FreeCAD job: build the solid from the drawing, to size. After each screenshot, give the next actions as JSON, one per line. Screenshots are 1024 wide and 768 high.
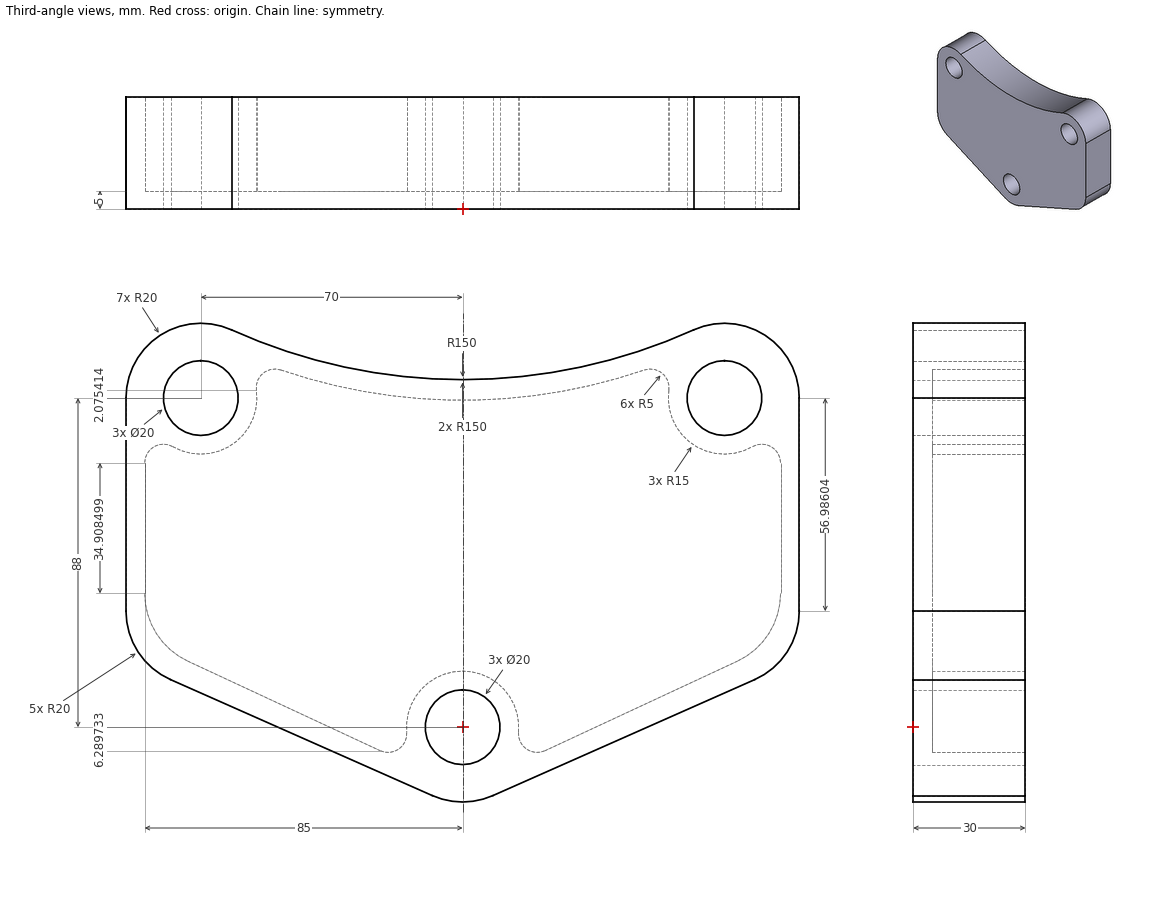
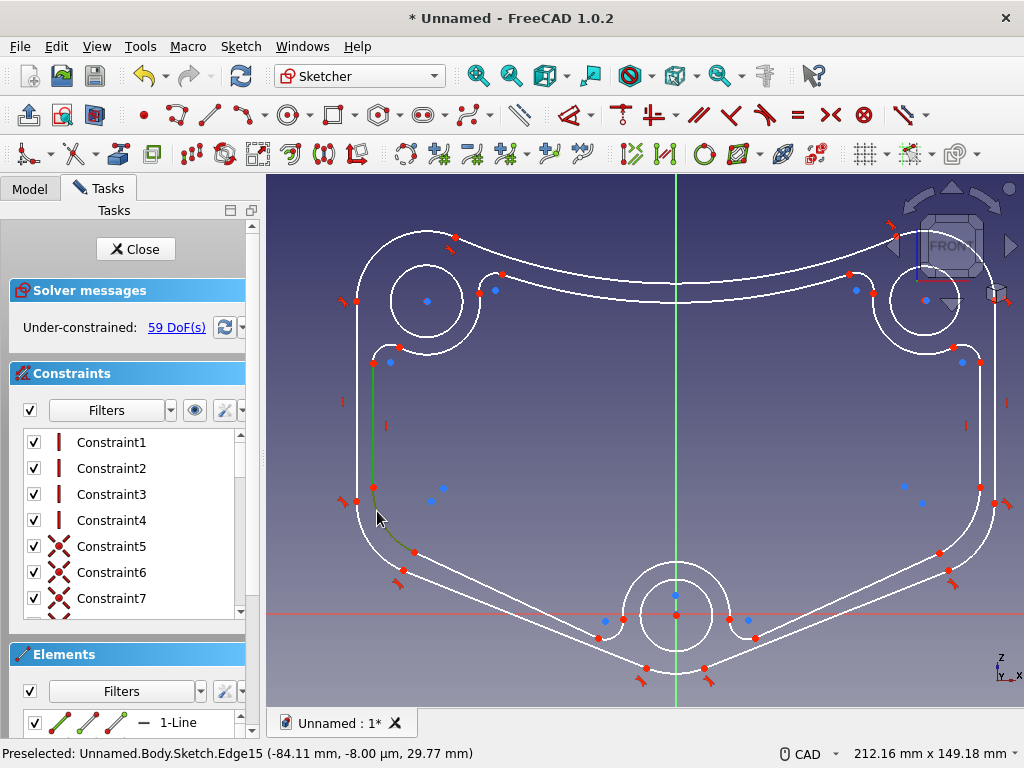
{"action": "left_click", "coordinate": [765, 116]}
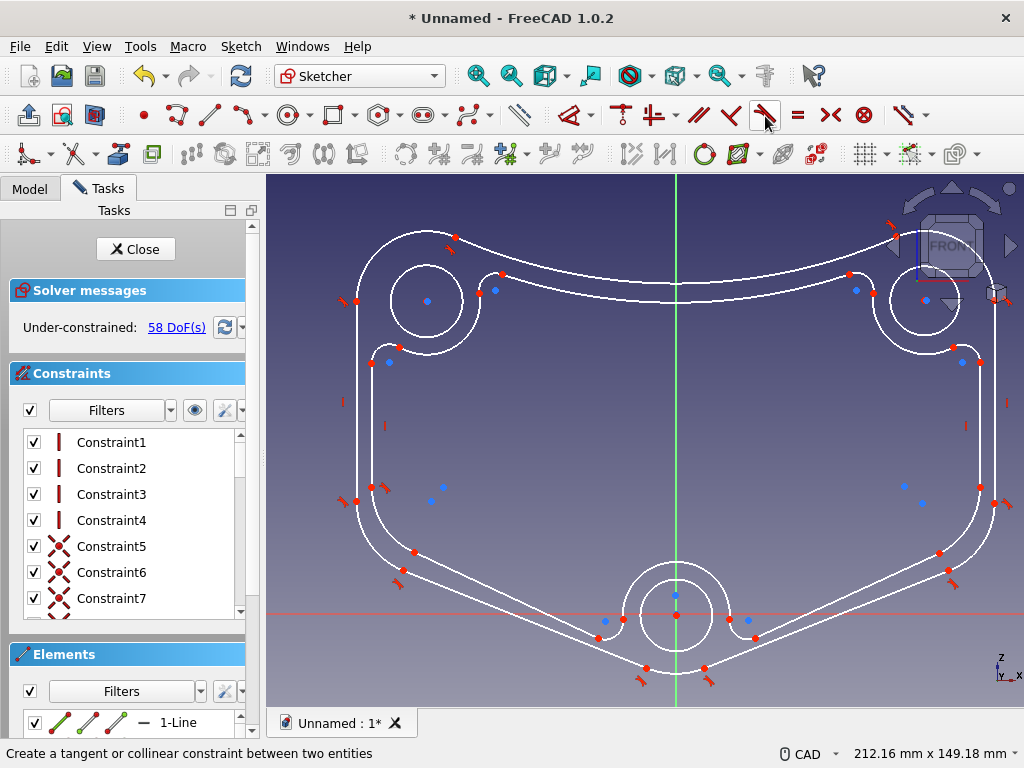
{"action": "left_click", "coordinate": [372, 400]}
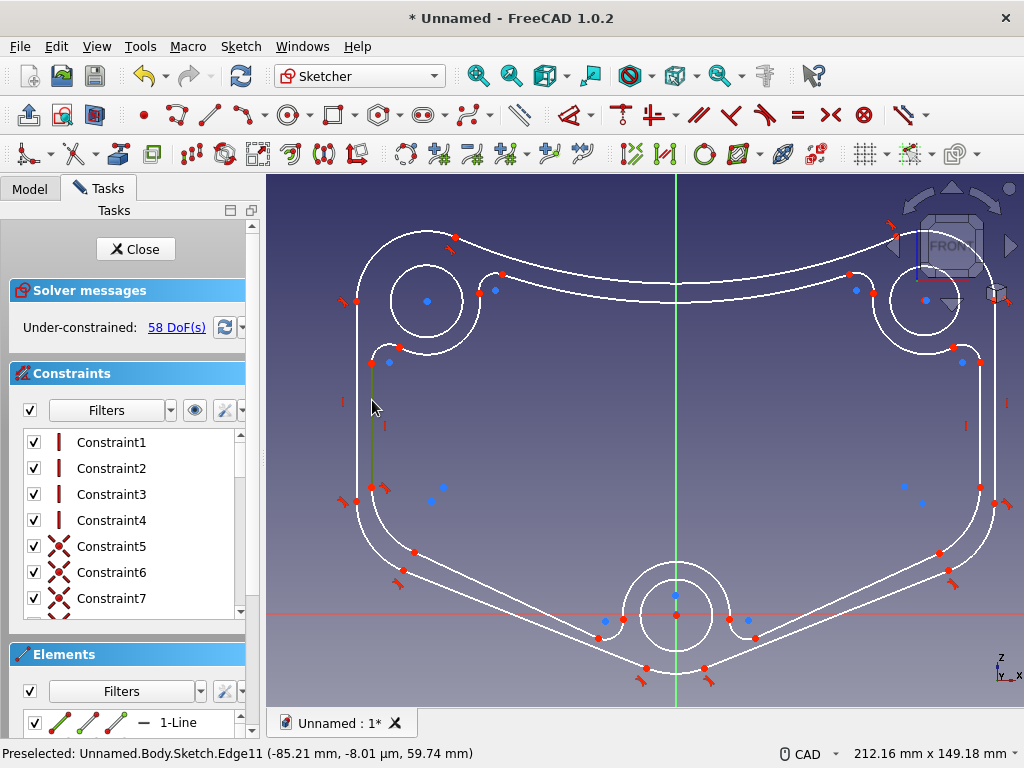
{"action": "left_click", "coordinate": [388, 344]}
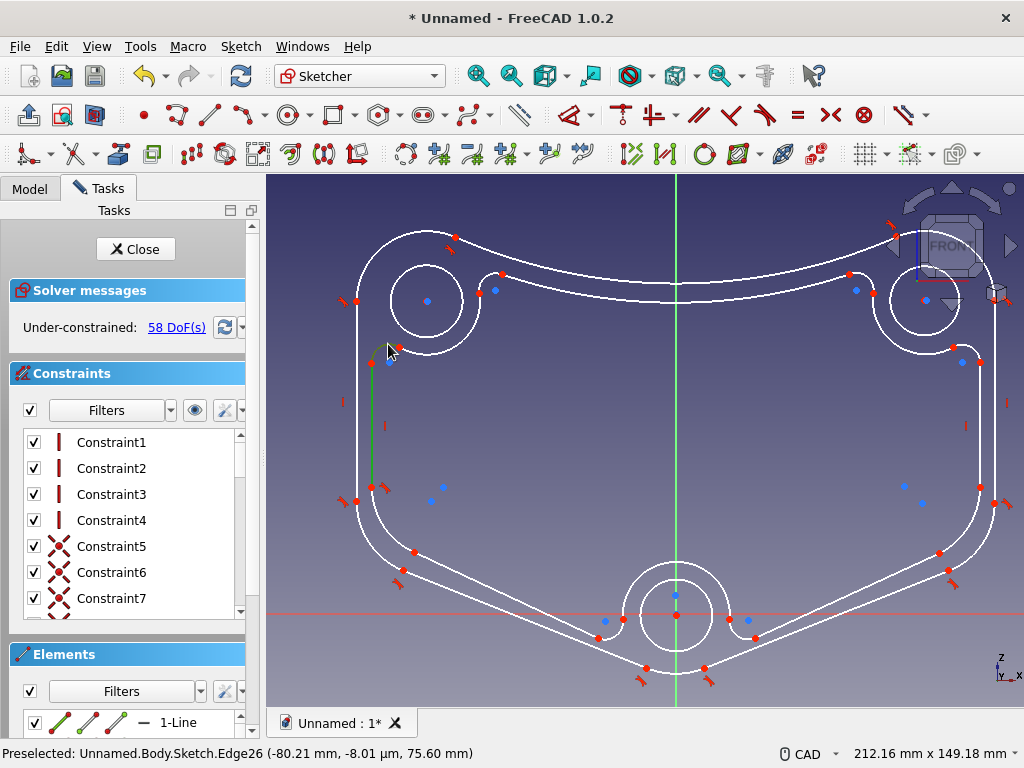
{"action": "left_click", "coordinate": [765, 116]}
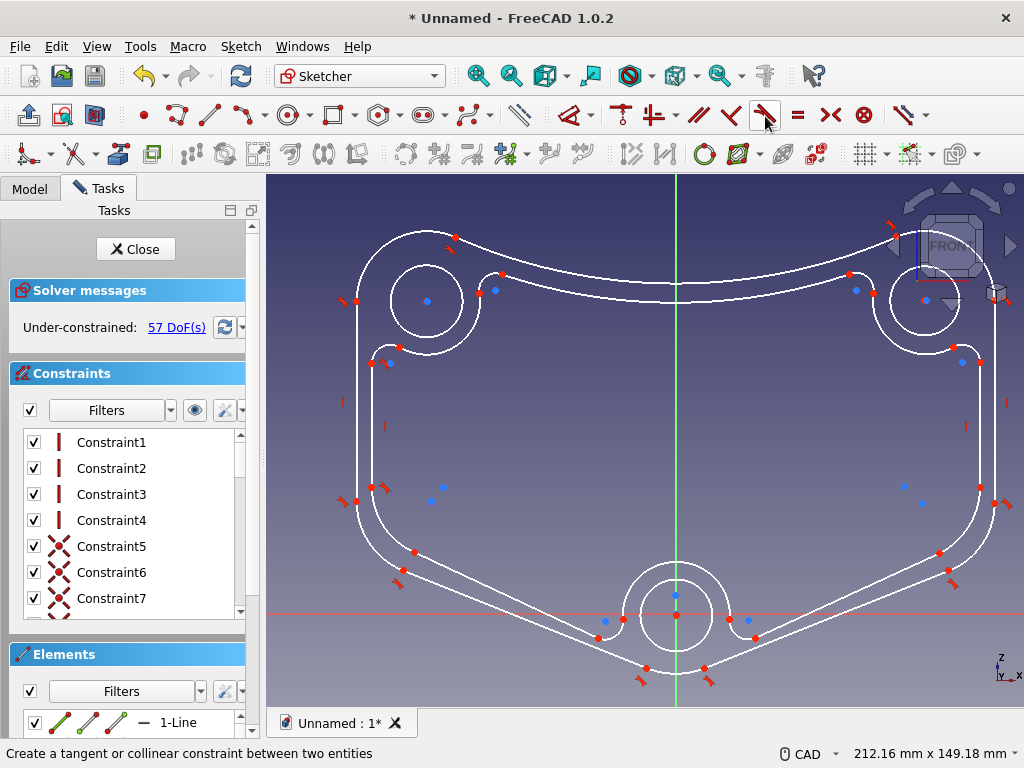
{"action": "left_click", "coordinate": [469, 578]}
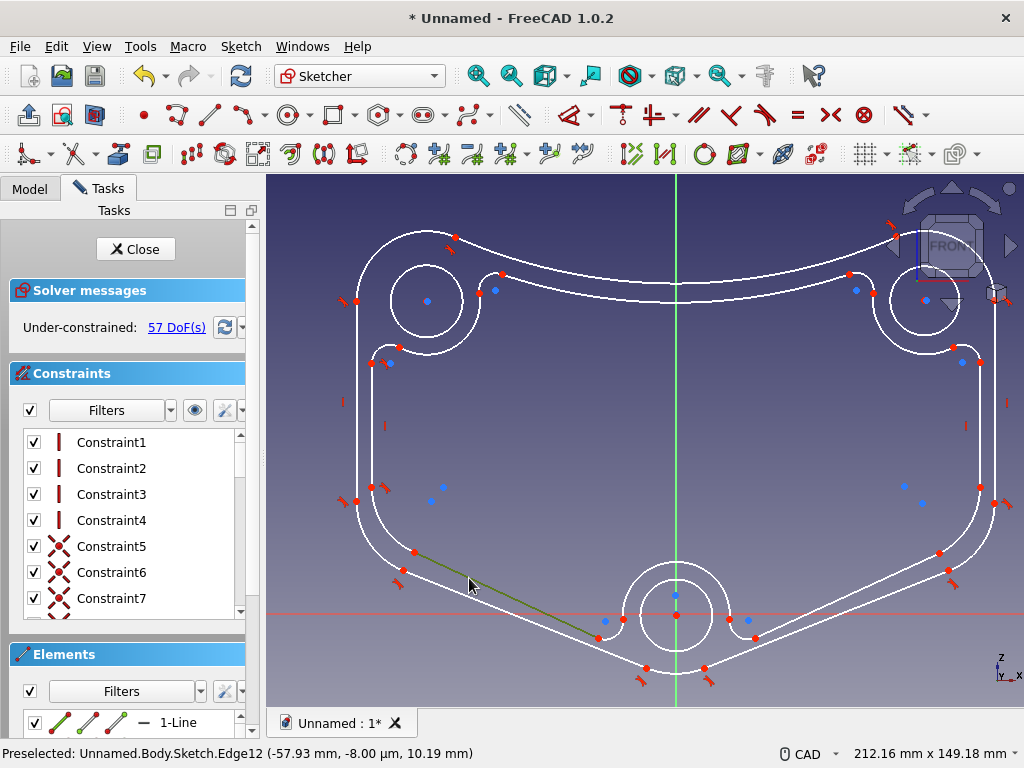
{"action": "left_click", "coordinate": [376, 511]}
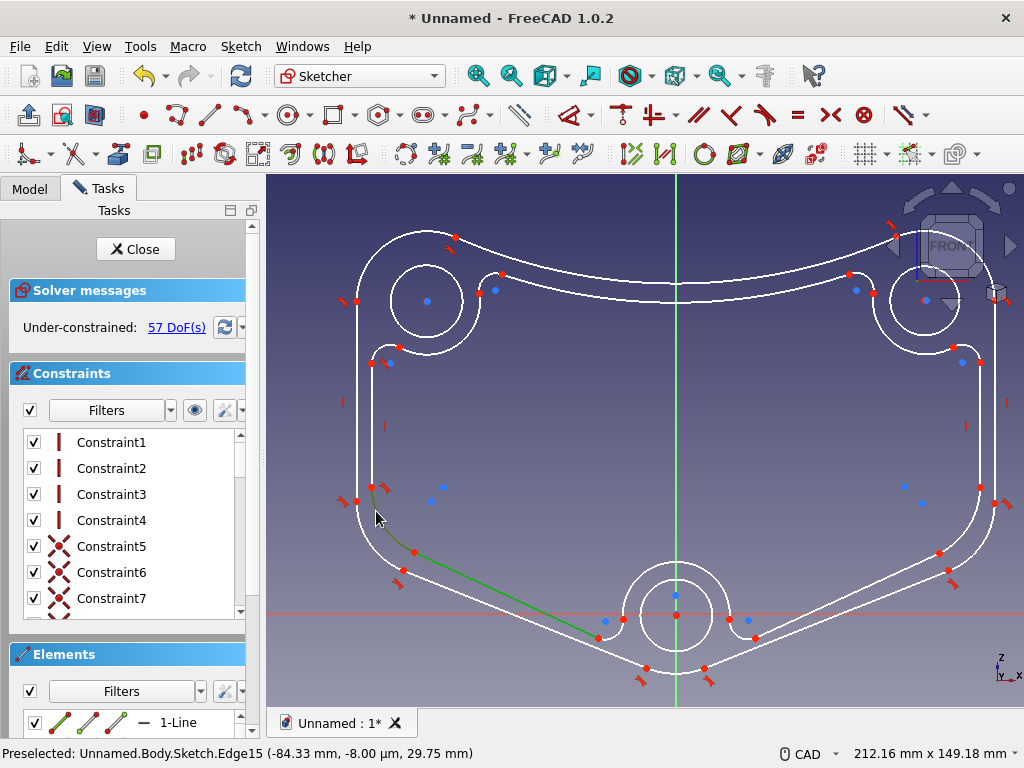
{"action": "key", "text": "t"}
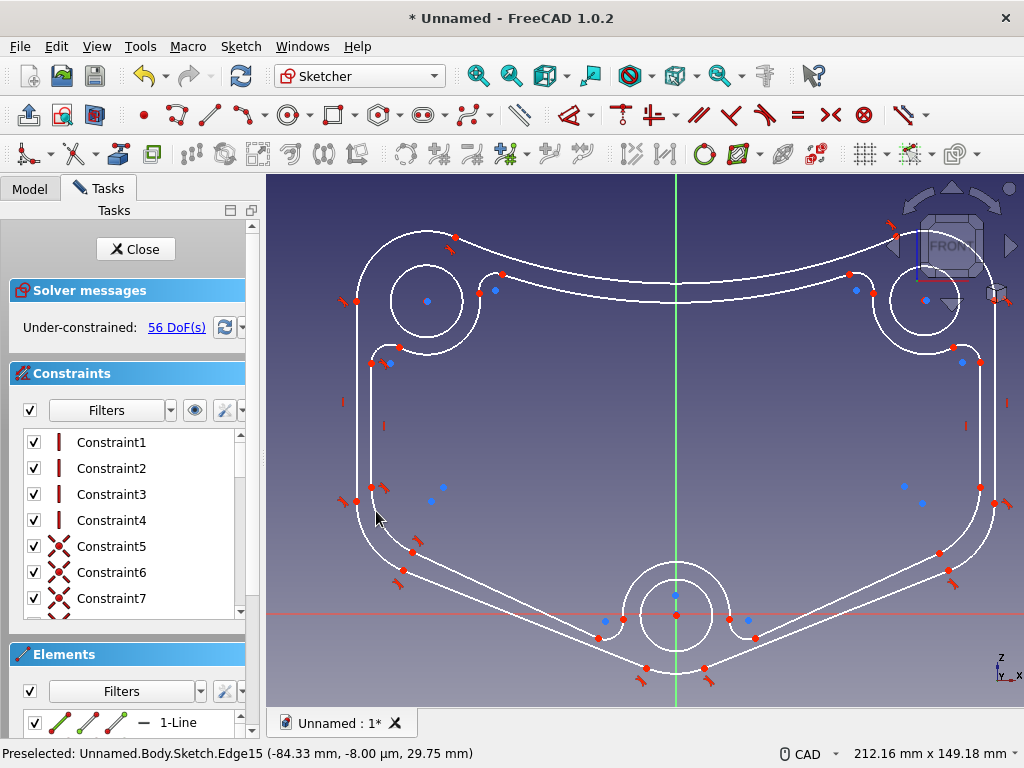
{"action": "left_click", "coordinate": [469, 578]}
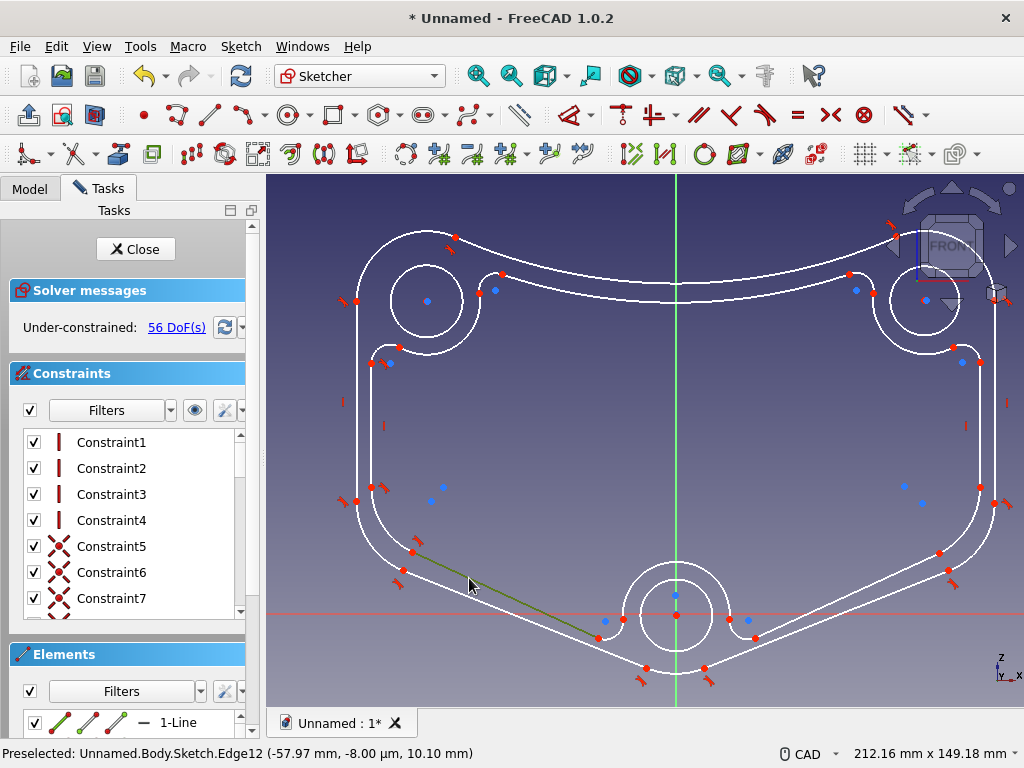
{"action": "scroll", "coordinate": [609, 639], "scroll_direction": "up", "scroll_amount": 2}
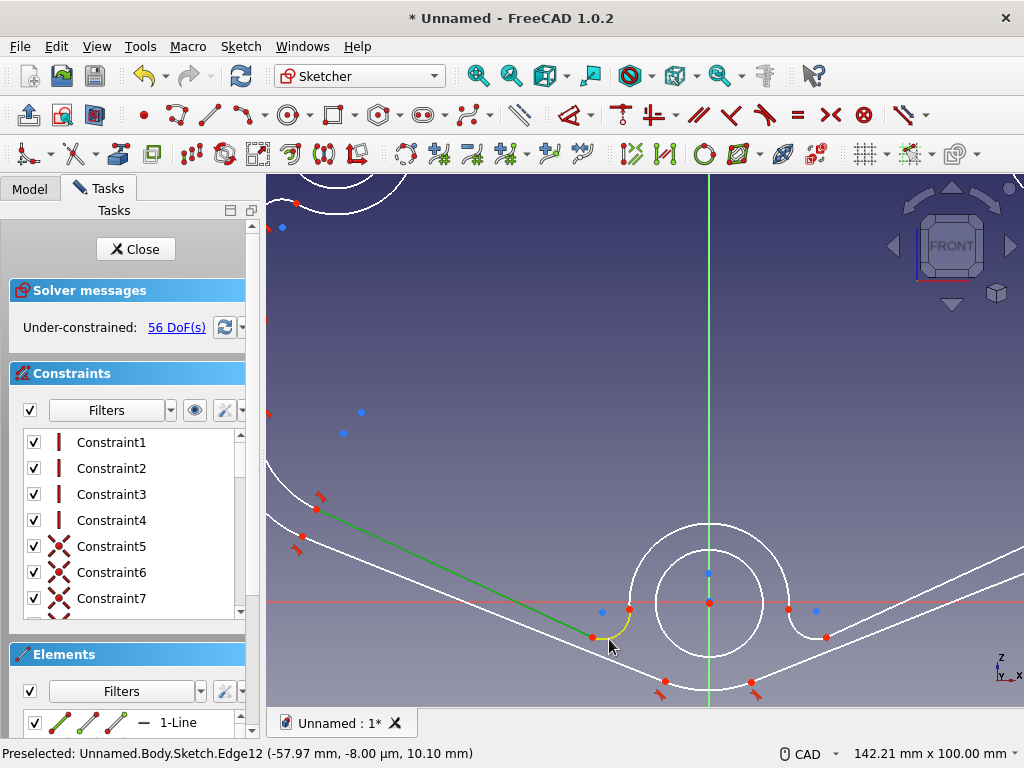
{"action": "left_click", "coordinate": [609, 639]}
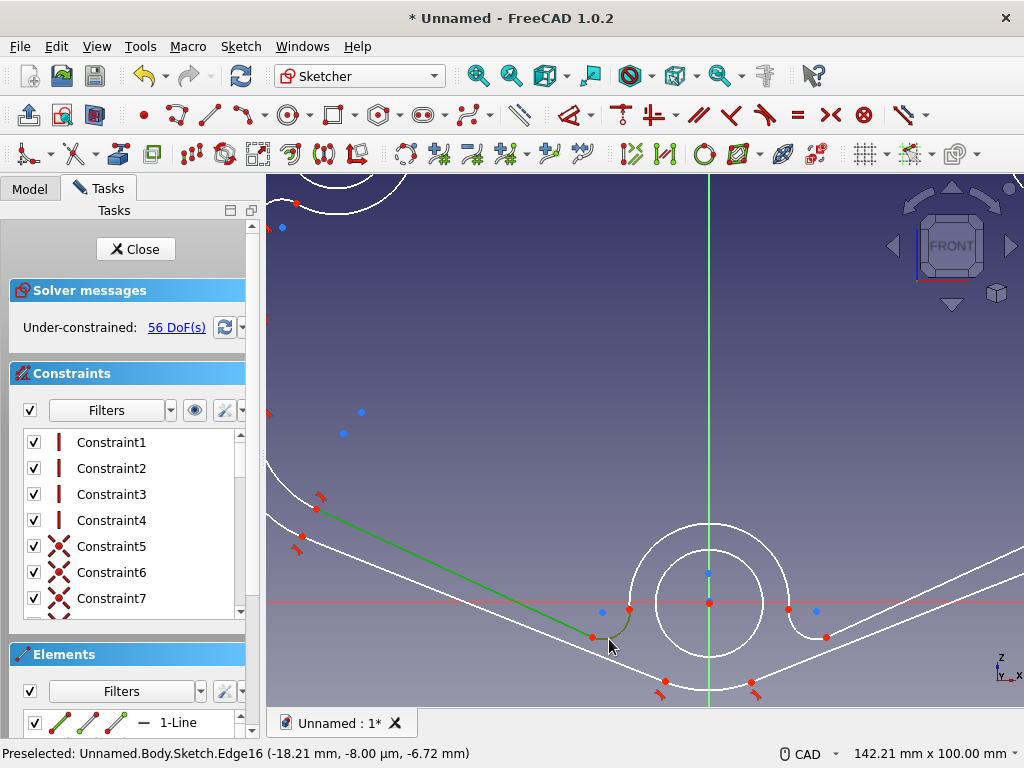
{"action": "left_click", "coordinate": [765, 116]}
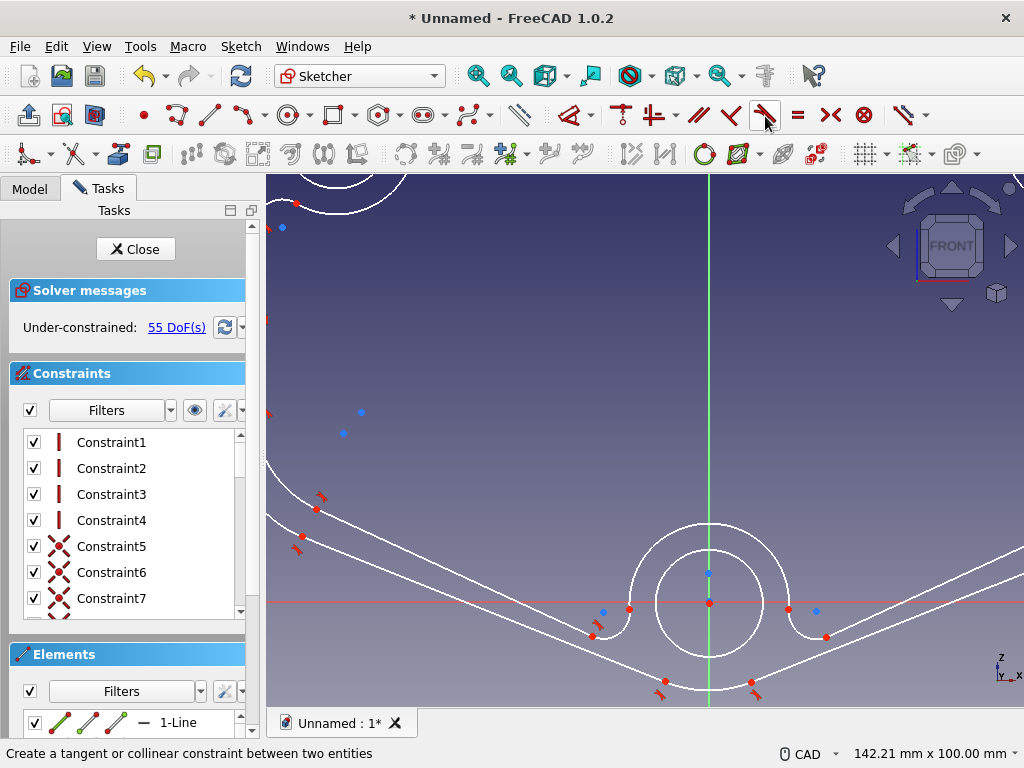
{"action": "scroll", "coordinate": [468, 496], "scroll_direction": "down", "scroll_amount": 4}